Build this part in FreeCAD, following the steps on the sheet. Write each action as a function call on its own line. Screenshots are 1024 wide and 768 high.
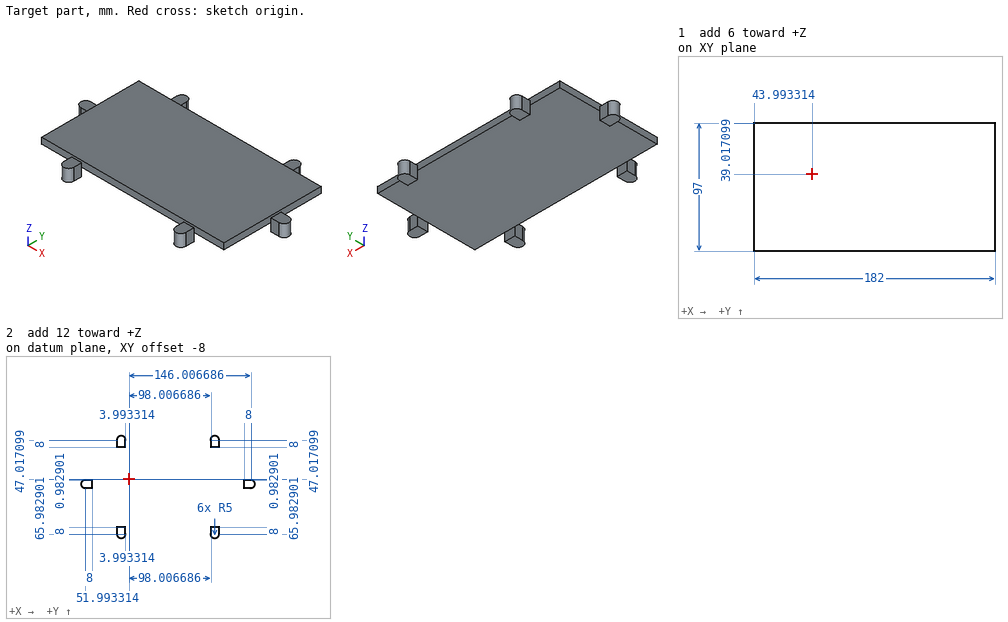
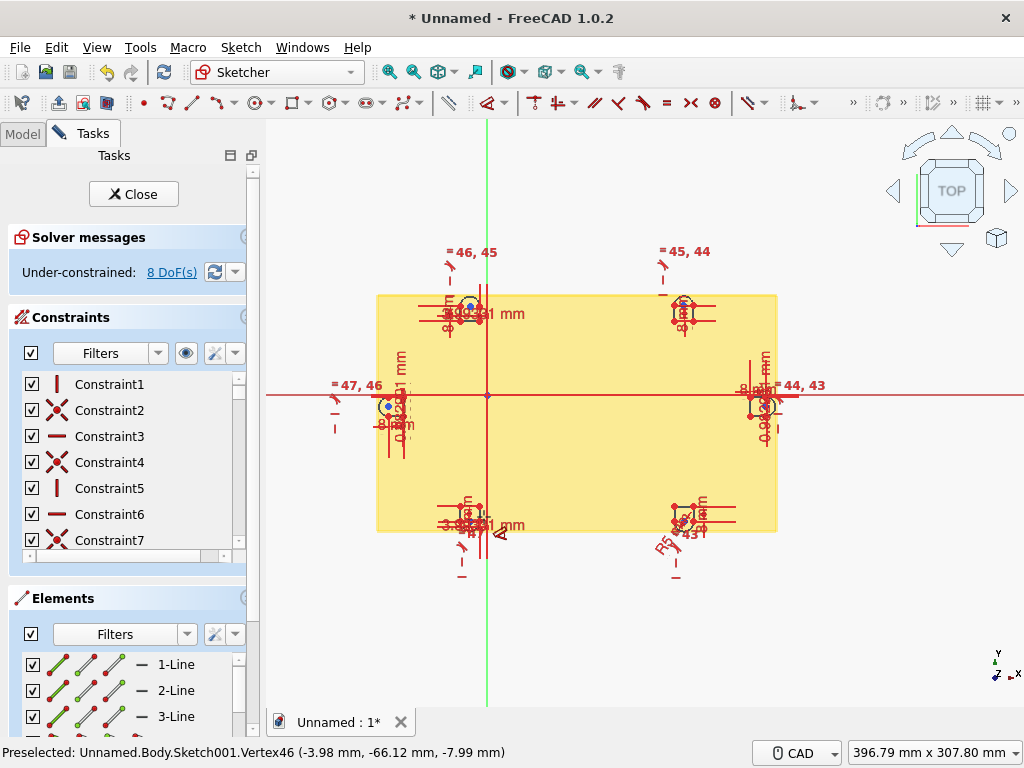
scroll(694, 522, up, 2)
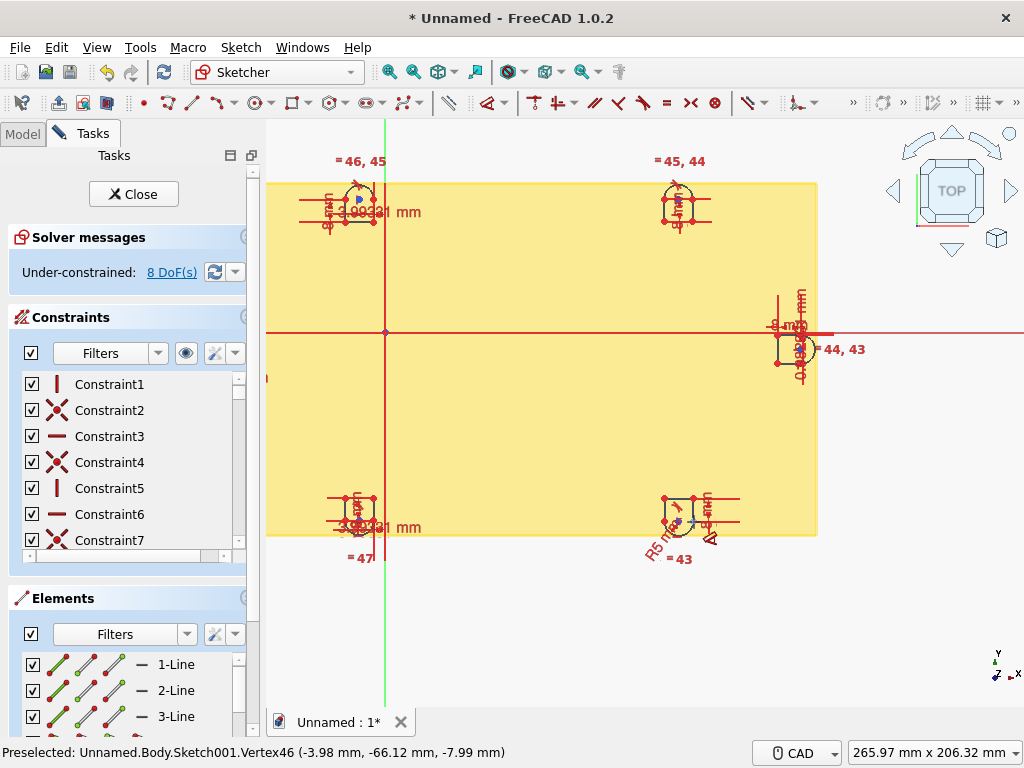
click(693, 522)
click(727, 427)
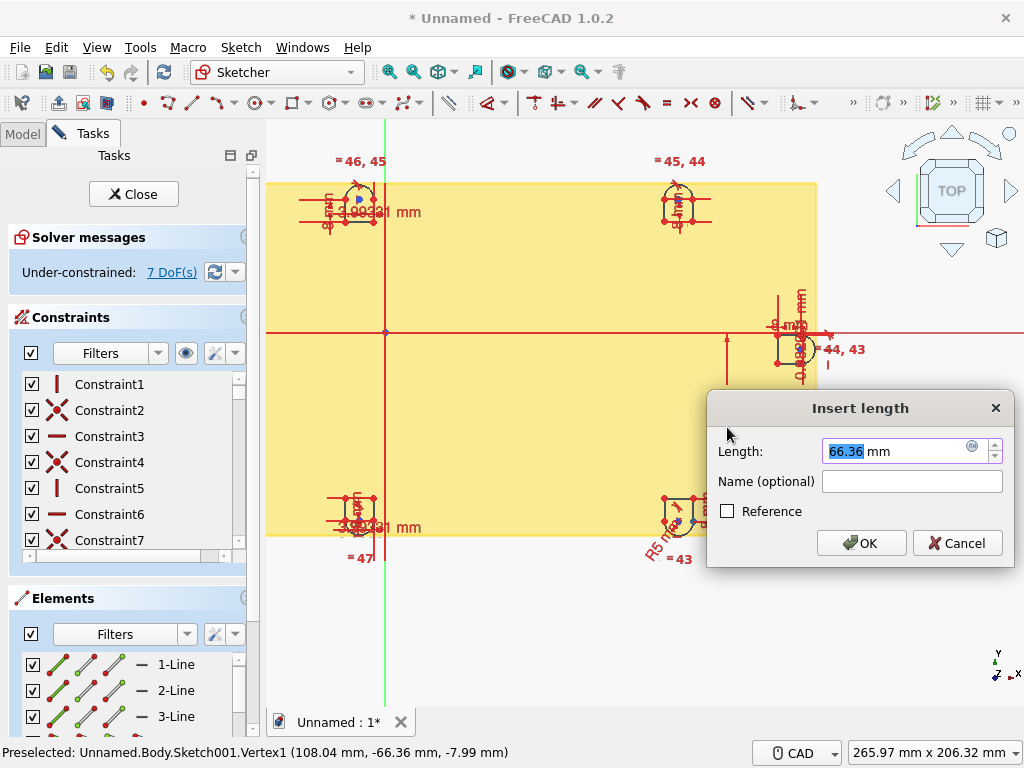
text(65.982901)
key(Return)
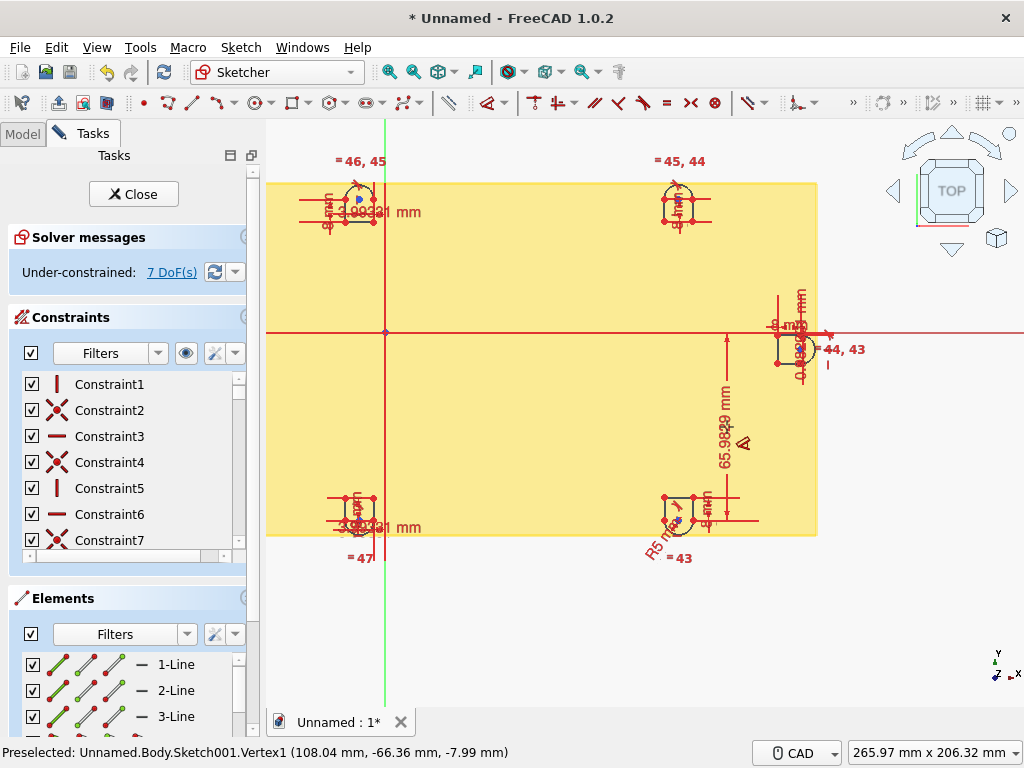
click(665, 498)
click(525, 532)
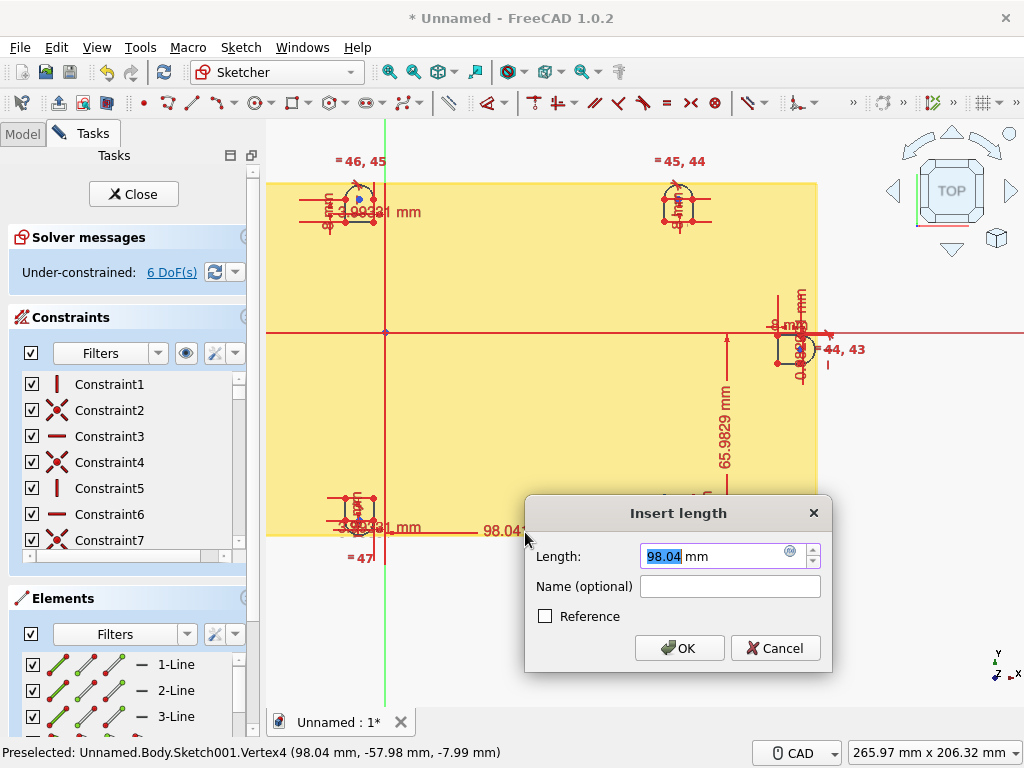
text(98.006686)
key(Return)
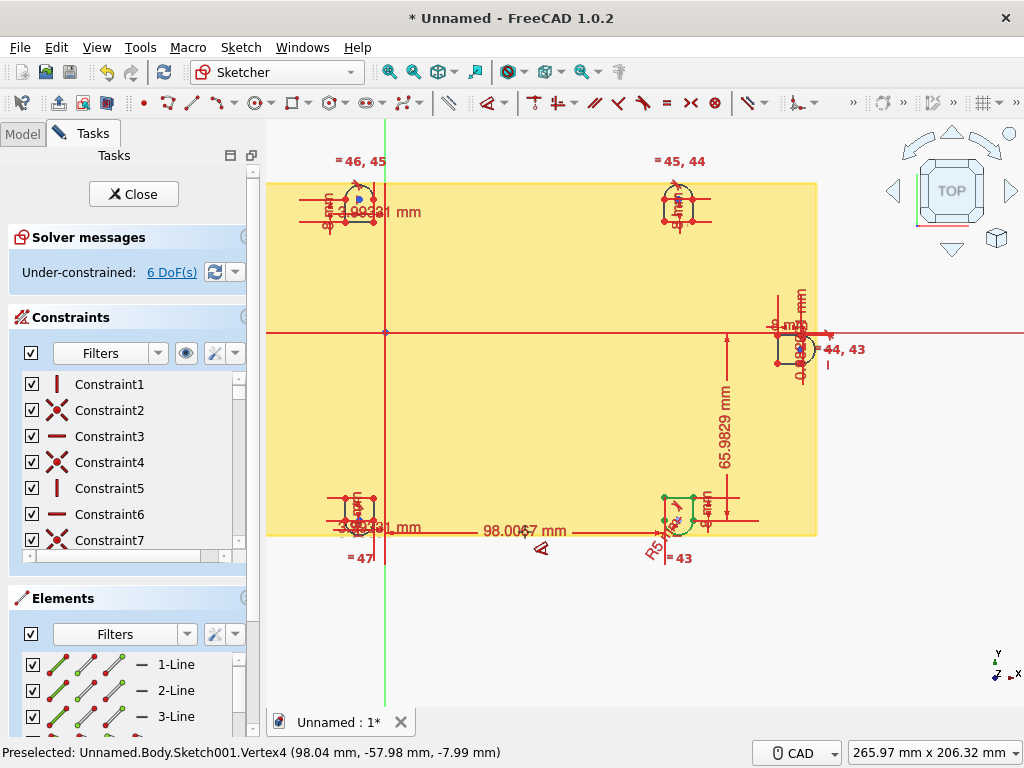
click(664, 199)
click(525, 165)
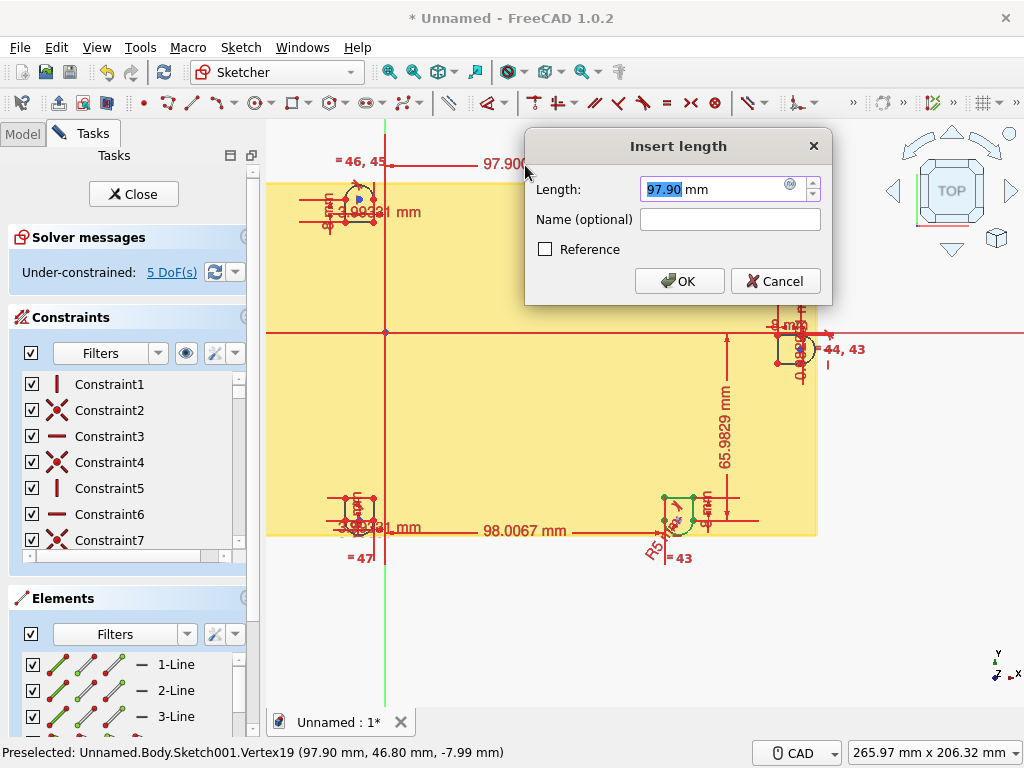
text(98.006686)
key(Return)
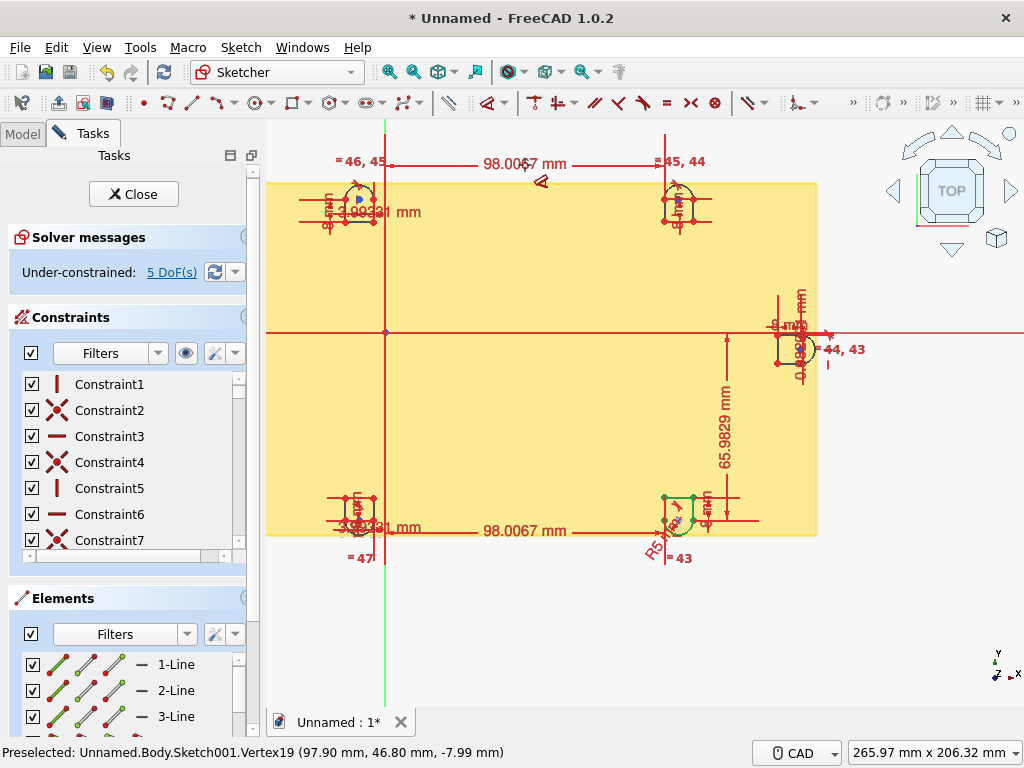
click(665, 199)
click(699, 266)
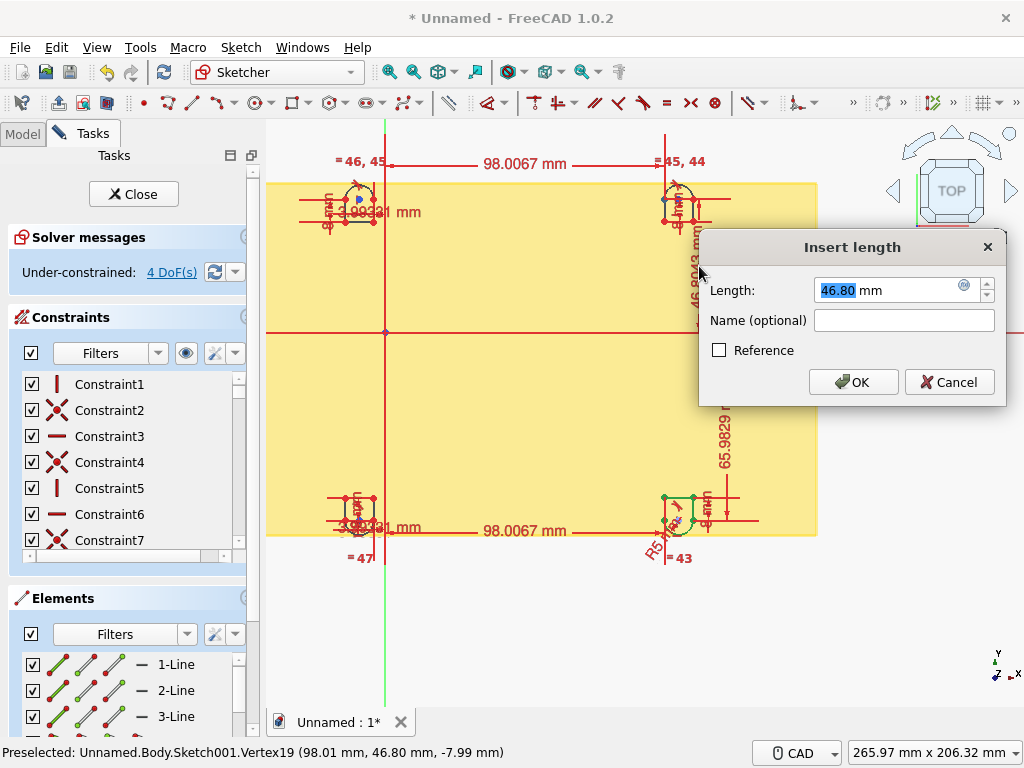
text(47.017099)
key(Return)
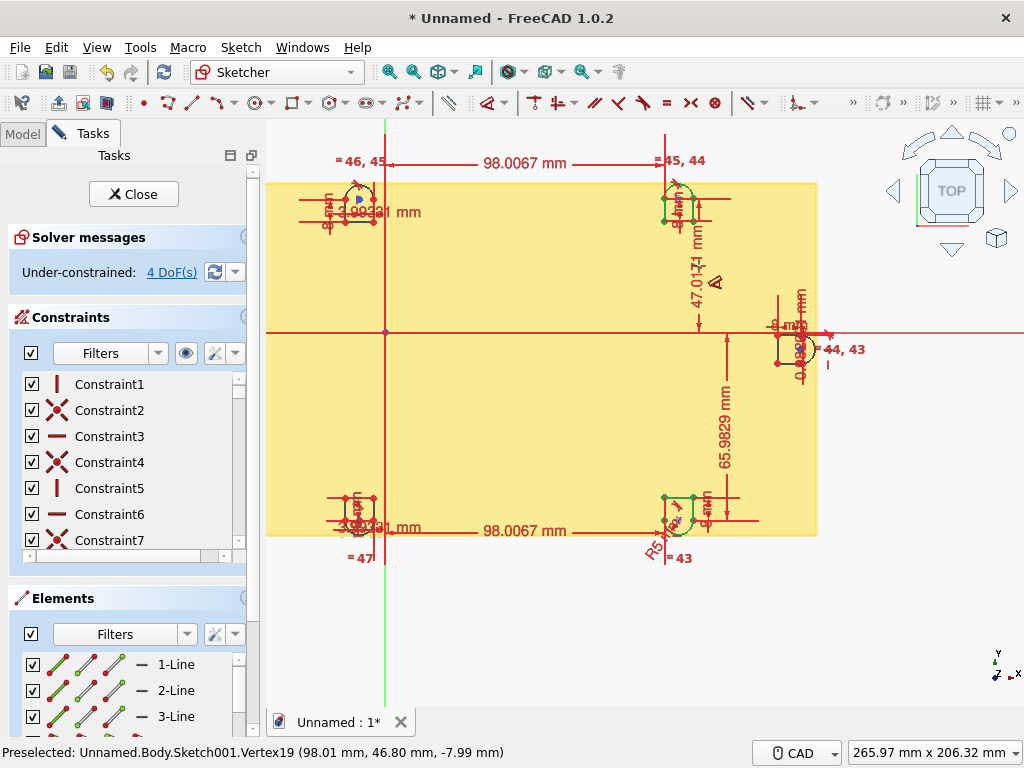
click(345, 200)
click(311, 266)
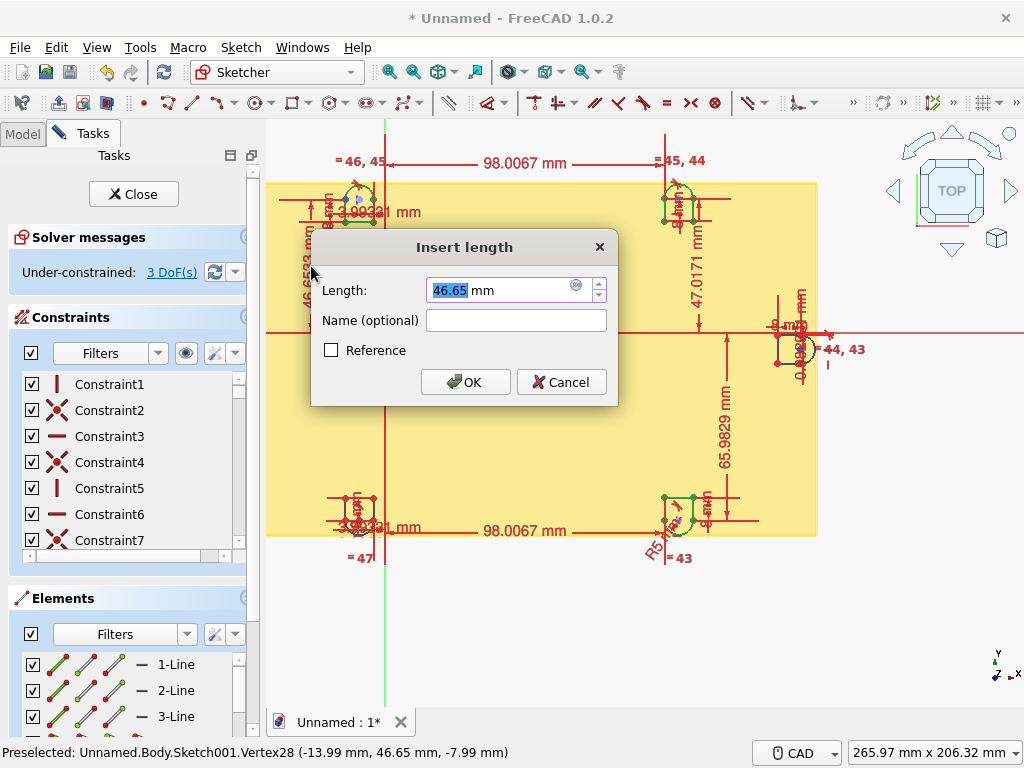
text(47.017099)
key(Return)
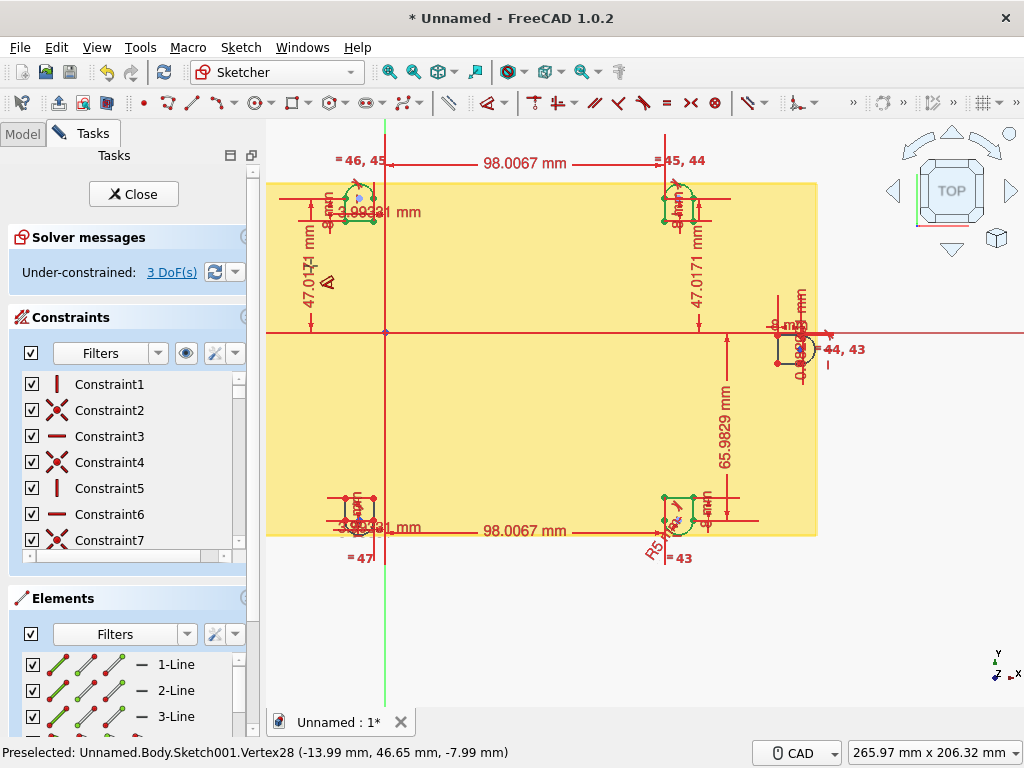
scroll(693, 522, down, 2)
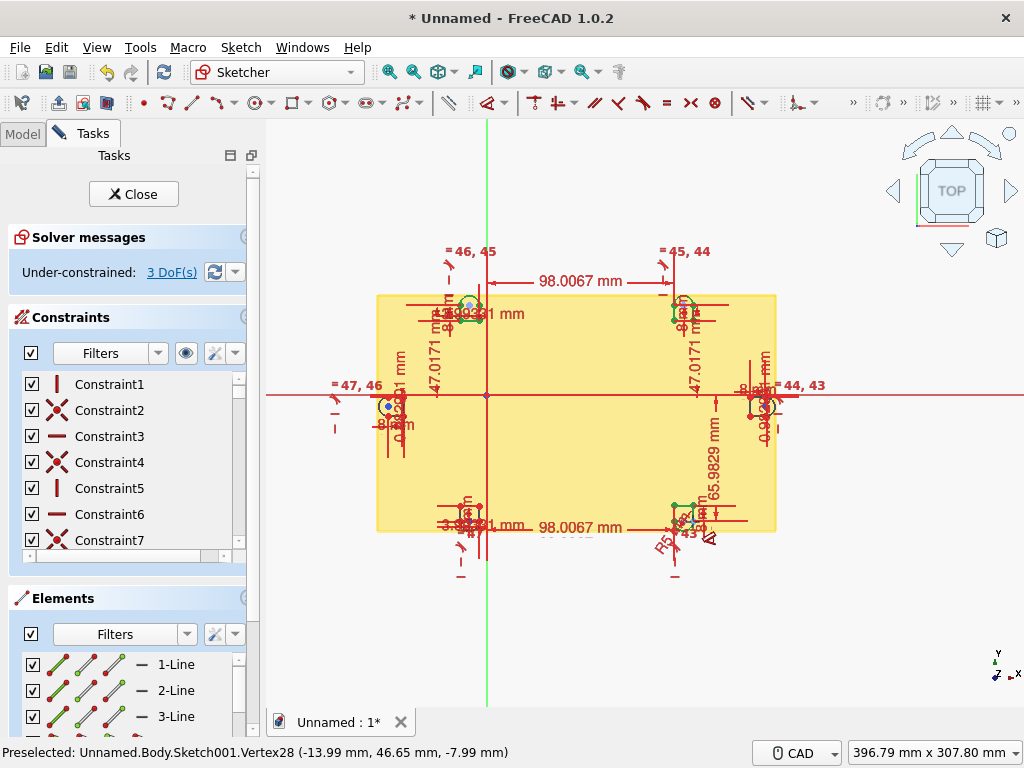
scroll(388, 416, up, 2)